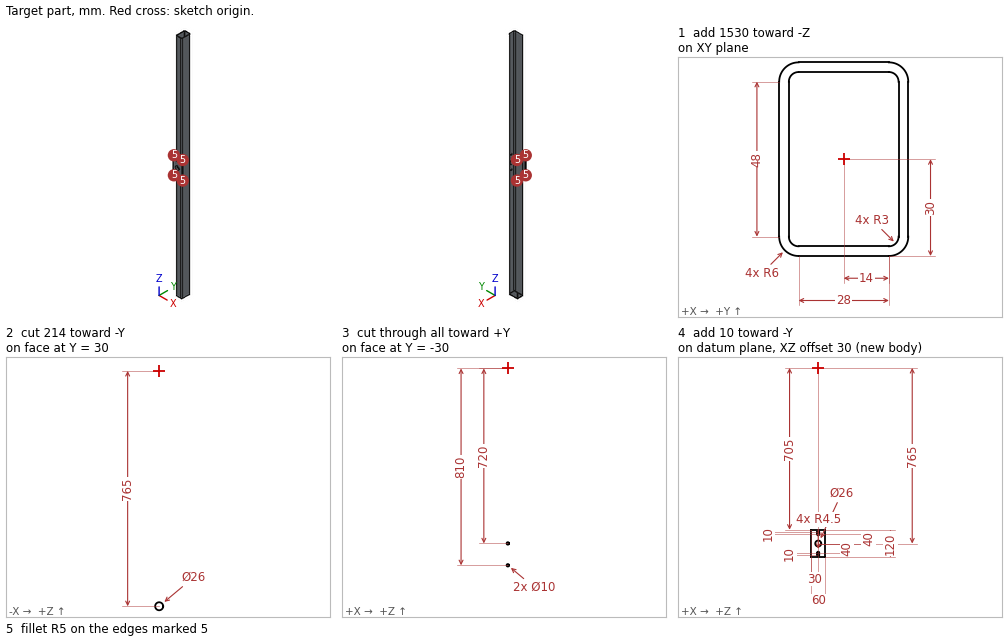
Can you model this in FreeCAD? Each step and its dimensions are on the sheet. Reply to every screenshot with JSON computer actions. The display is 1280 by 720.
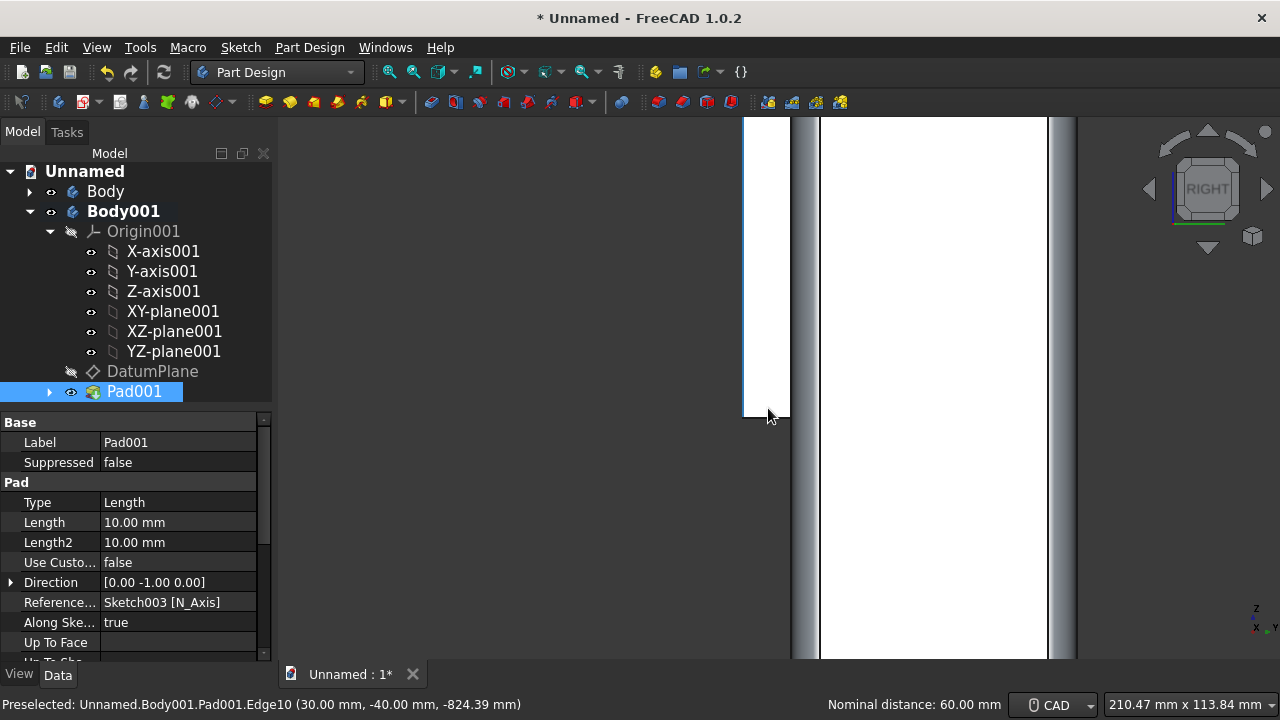
{"action": "left_click", "coordinate": [767, 417], "text": "ctrl"}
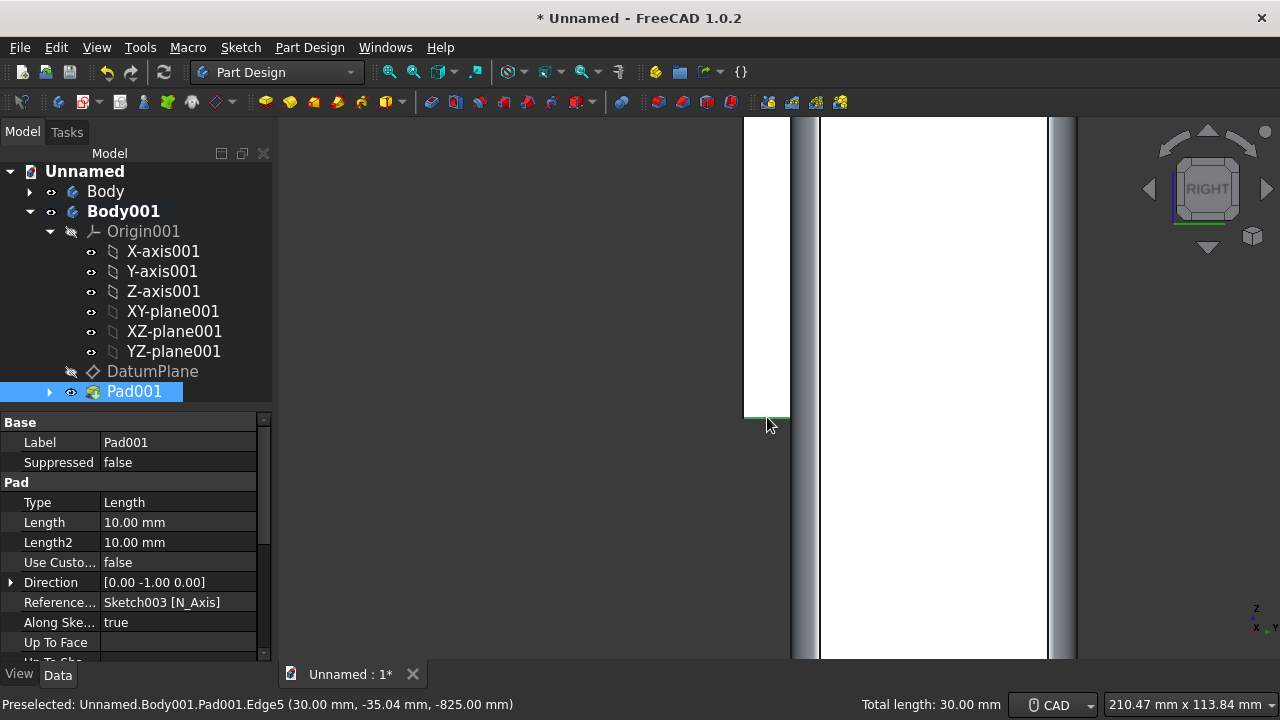
{"action": "left_click", "coordinate": [390, 72]}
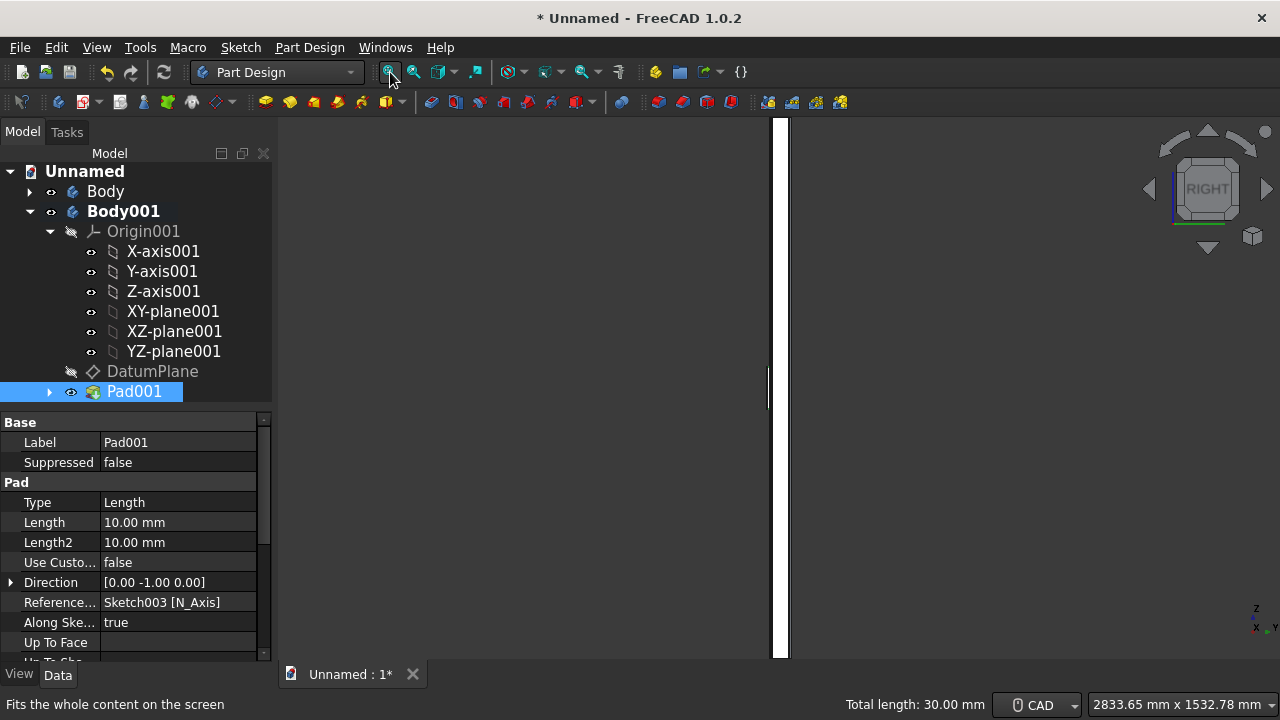
{"action": "key", "text": "5"}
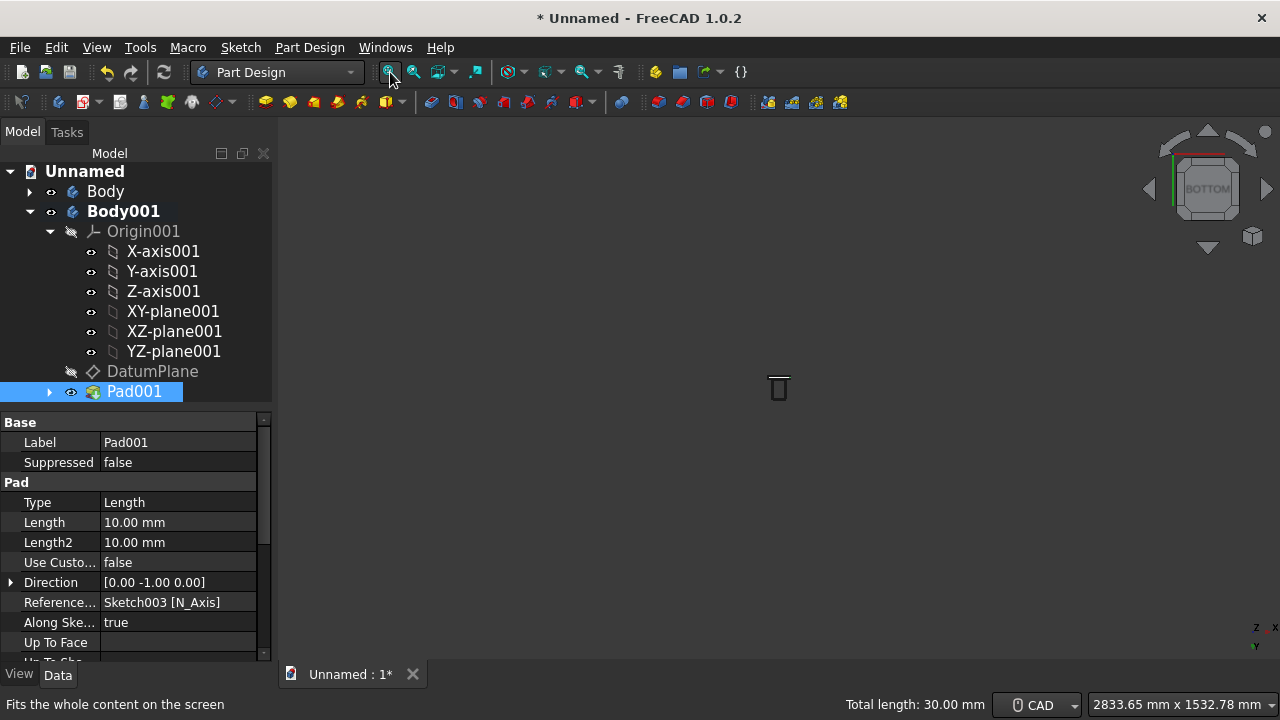
{"action": "left_click", "coordinate": [390, 72]}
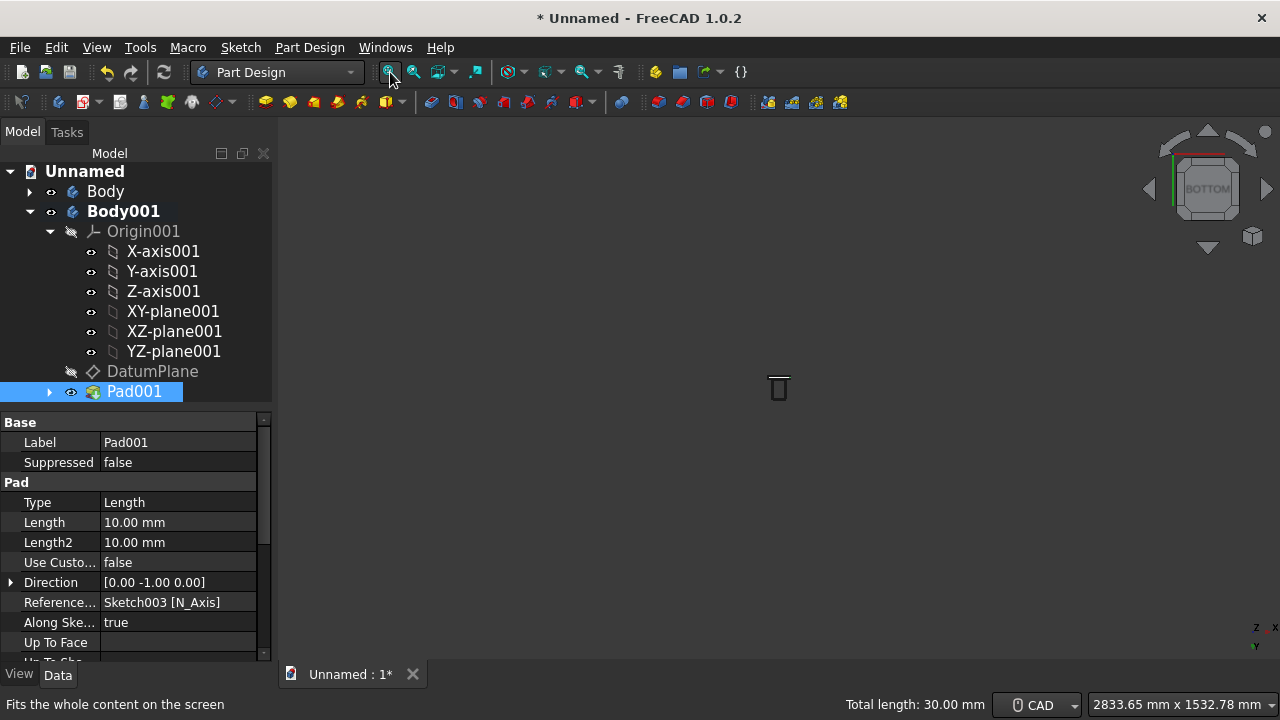
{"action": "scroll", "coordinate": [768, 376], "scroll_direction": "up", "scroll_amount": 13}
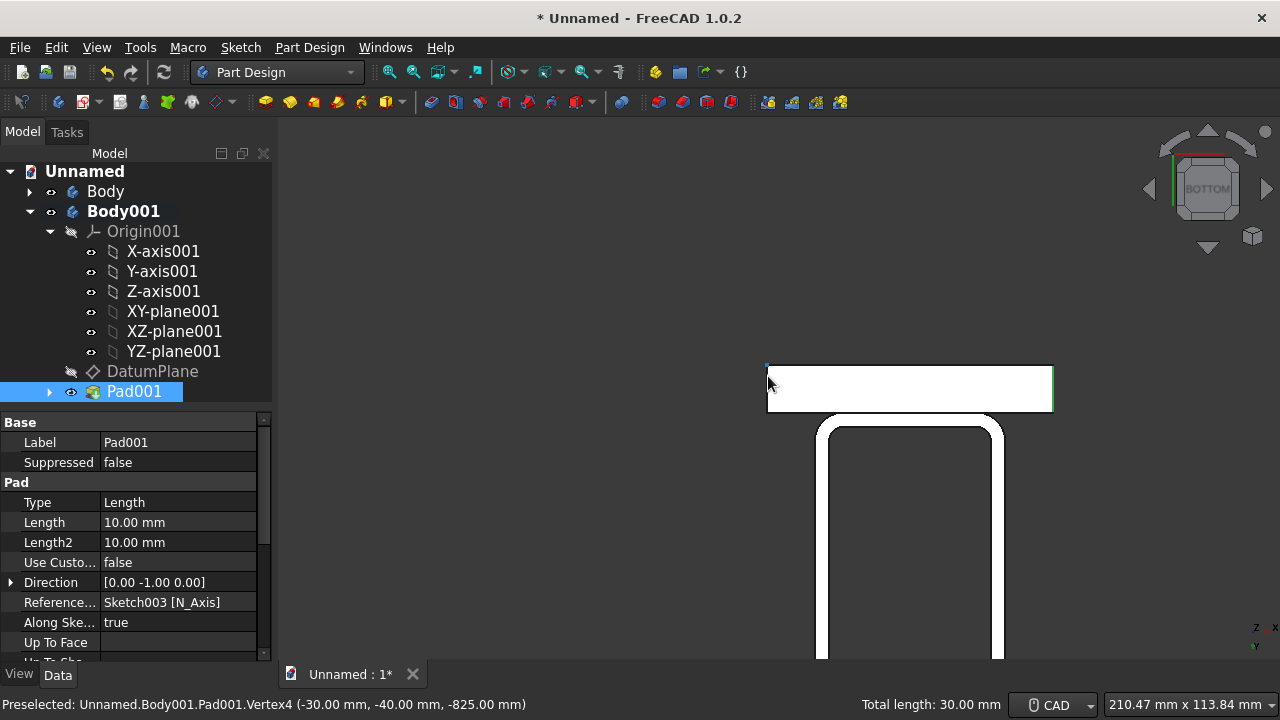
{"action": "left_click", "coordinate": [767, 388], "text": "ctrl"}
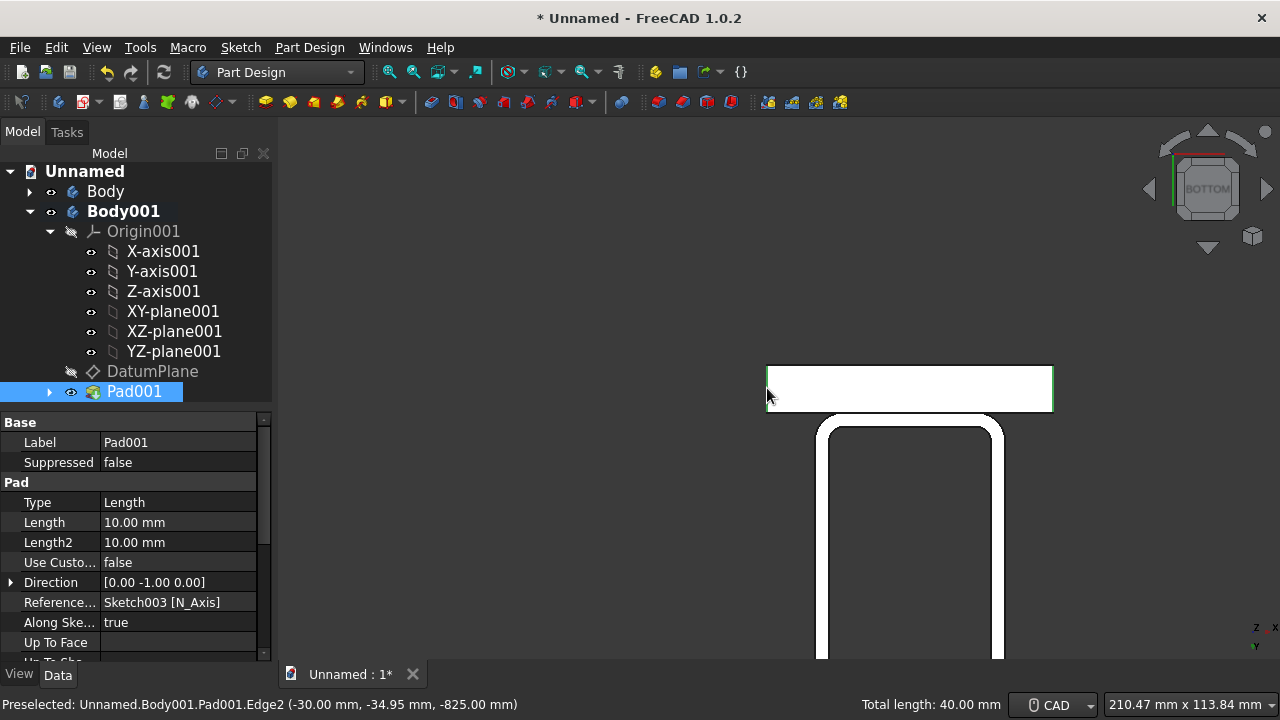
{"action": "left_click", "coordinate": [660, 102]}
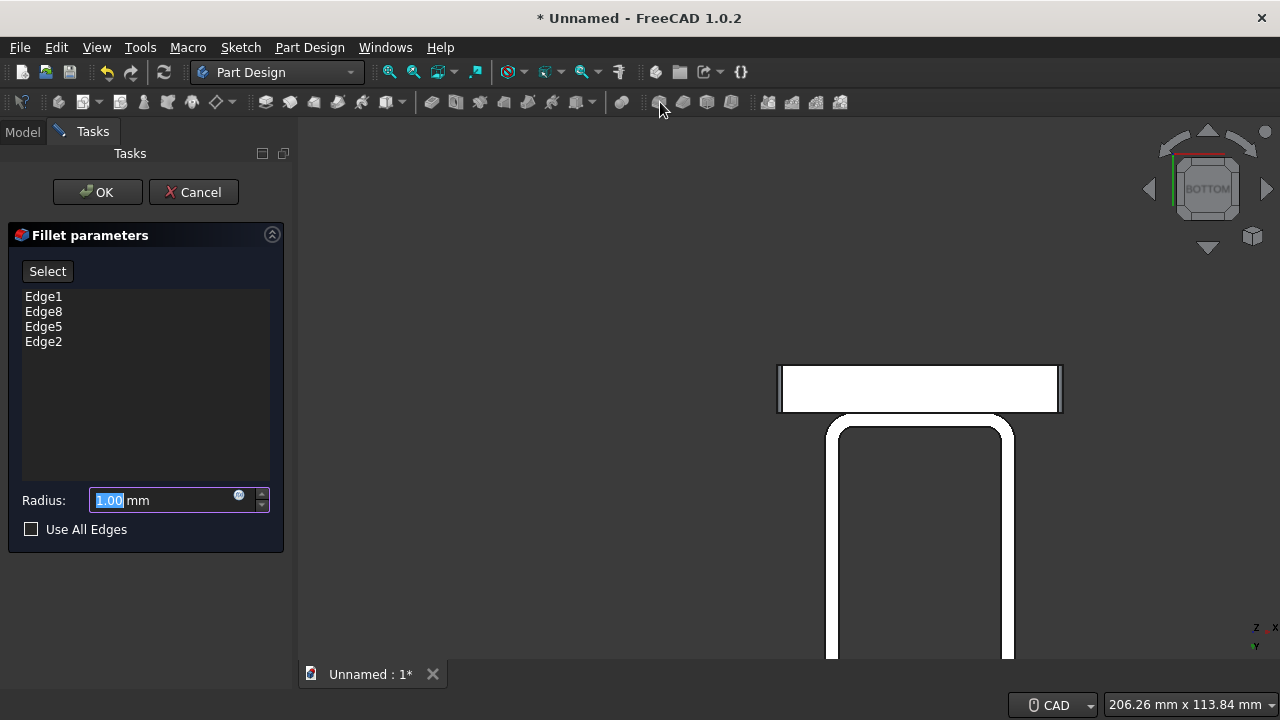
{"action": "type", "text": "5"}
{"action": "key", "text": "Tab"}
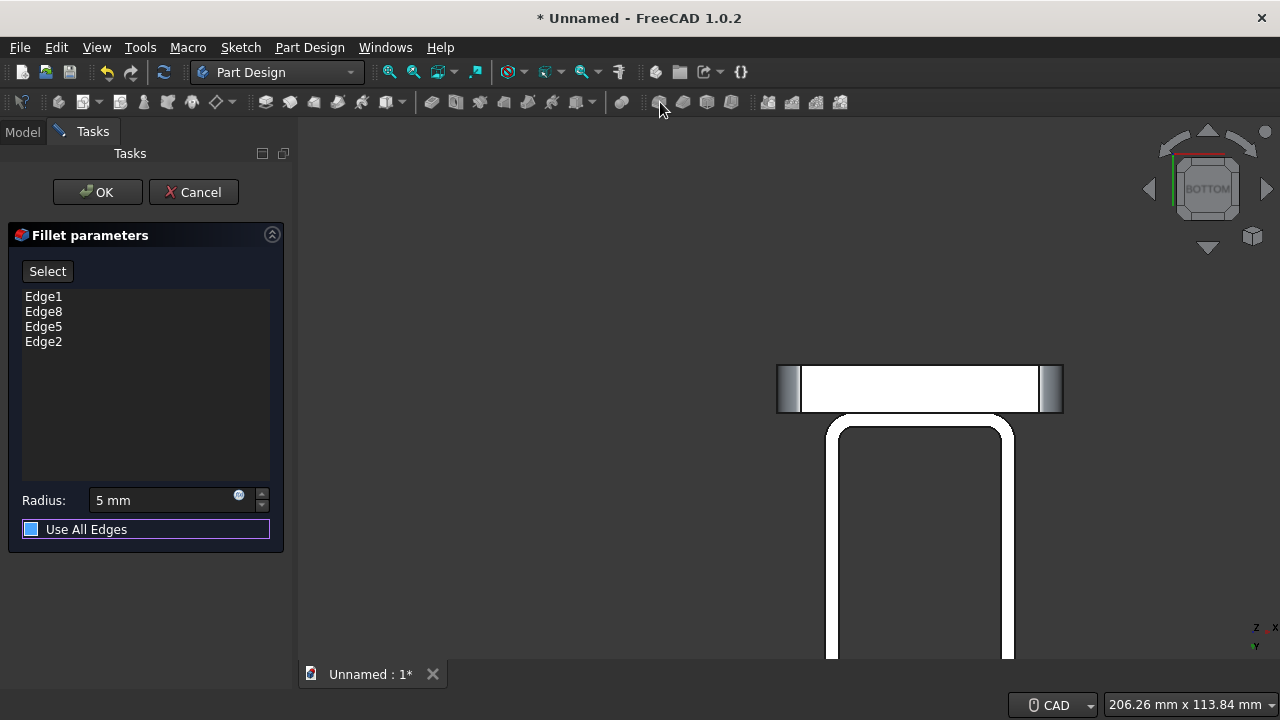
{"action": "left_click", "coordinate": [98, 192]}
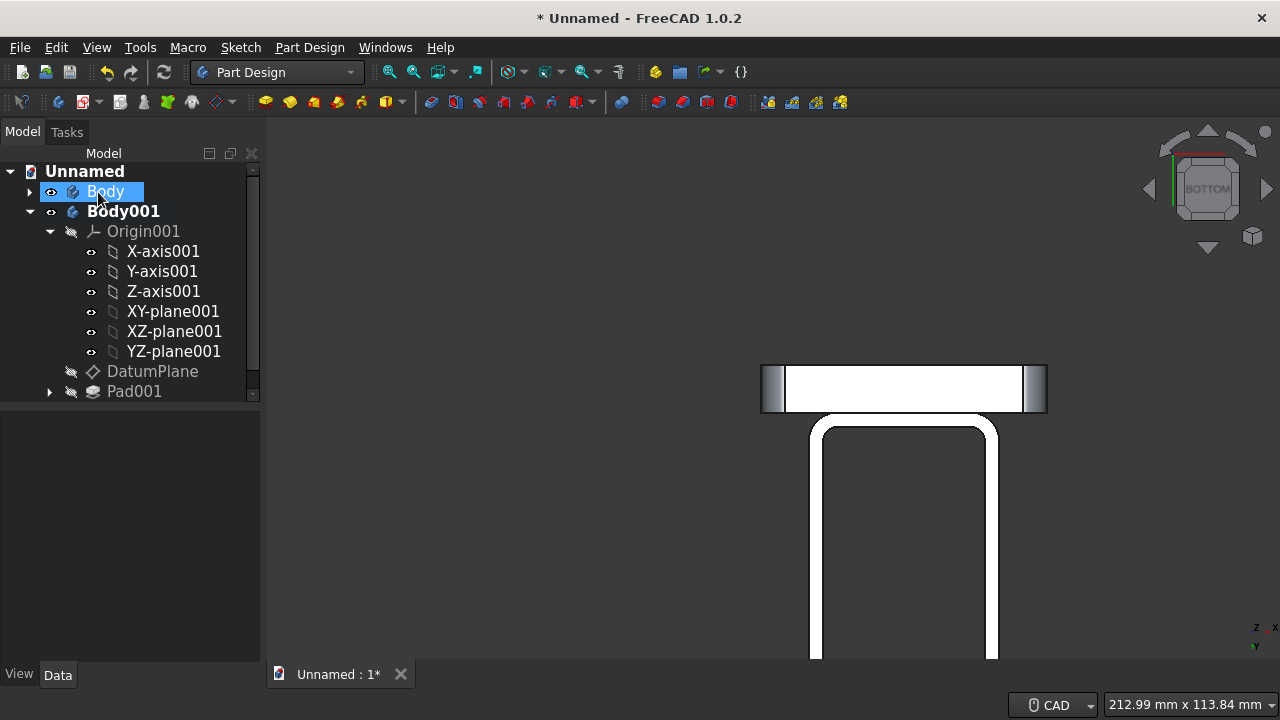
{"action": "key", "text": "0"}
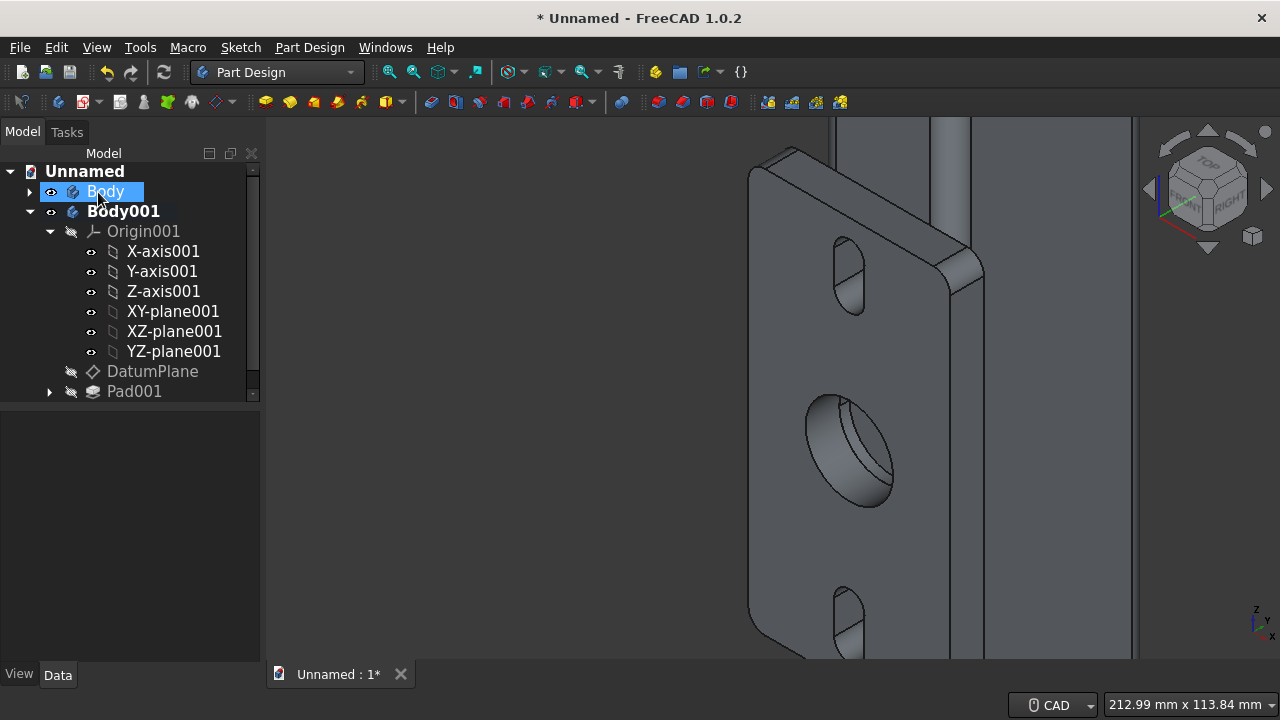
{"action": "left_click", "coordinate": [390, 72]}